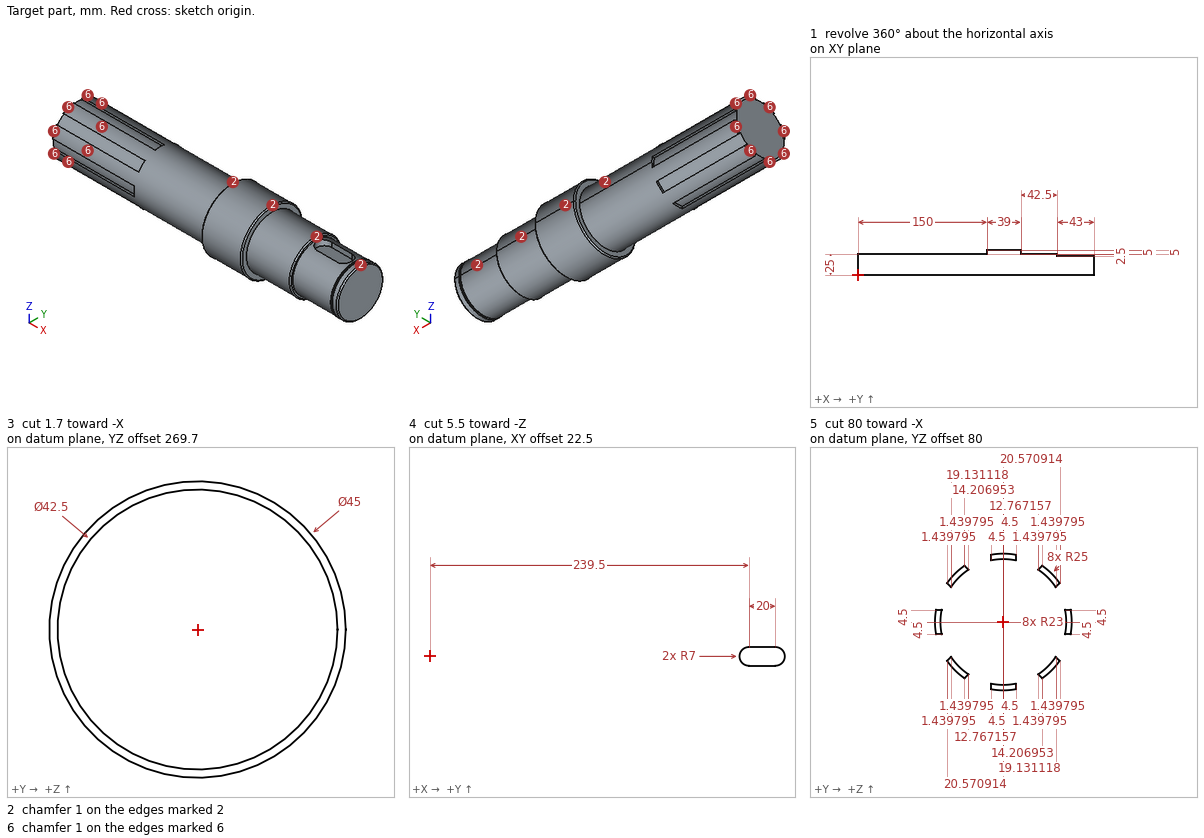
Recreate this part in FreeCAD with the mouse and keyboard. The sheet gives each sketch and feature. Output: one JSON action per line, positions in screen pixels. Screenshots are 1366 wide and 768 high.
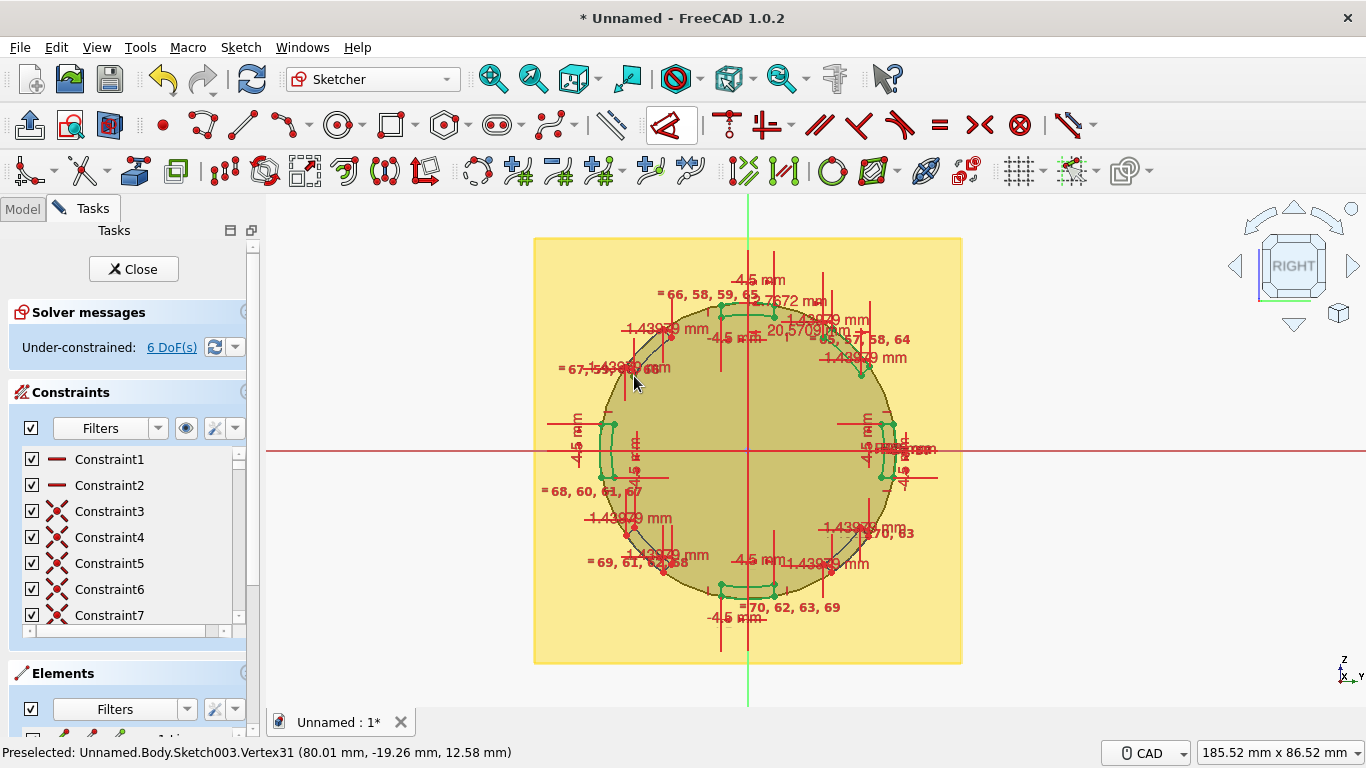
{"action": "left_click", "coordinate": [692, 126]}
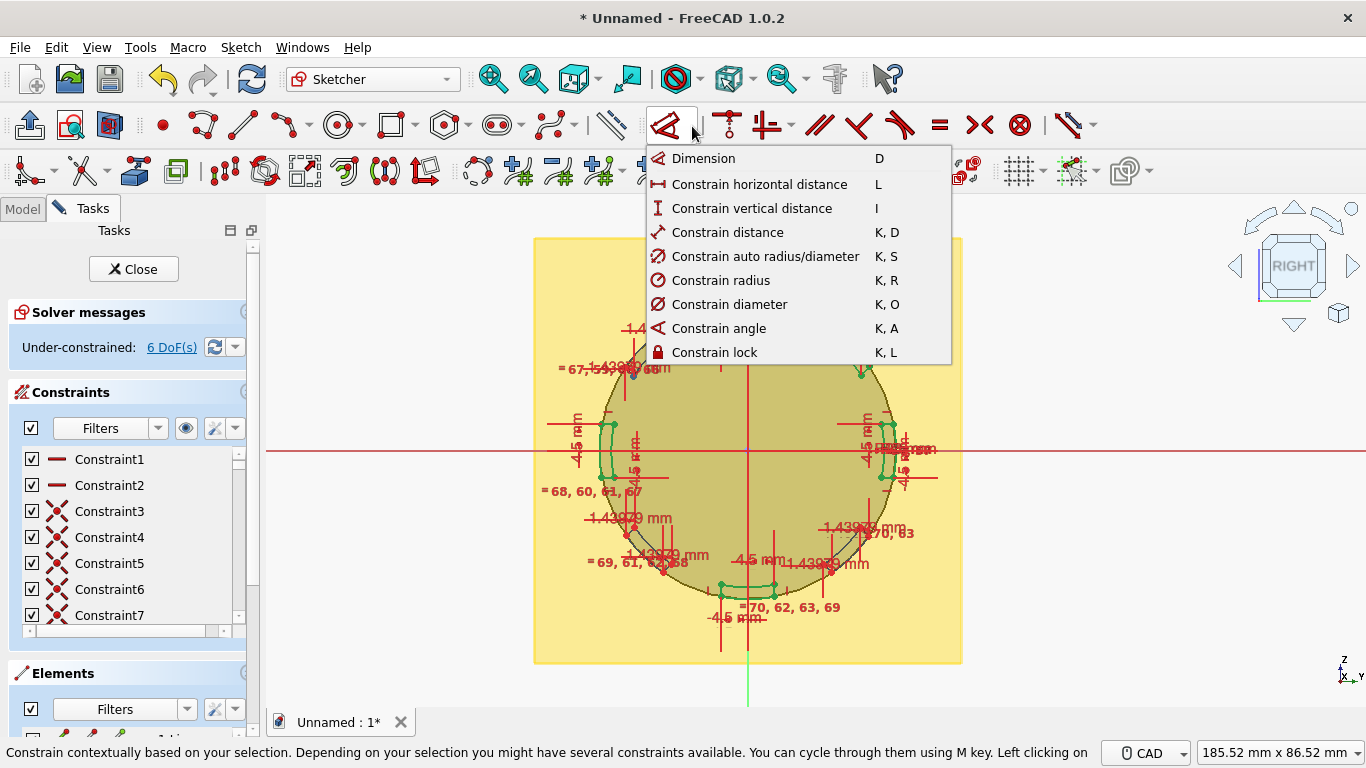
{"action": "left_click", "coordinate": [799, 184]}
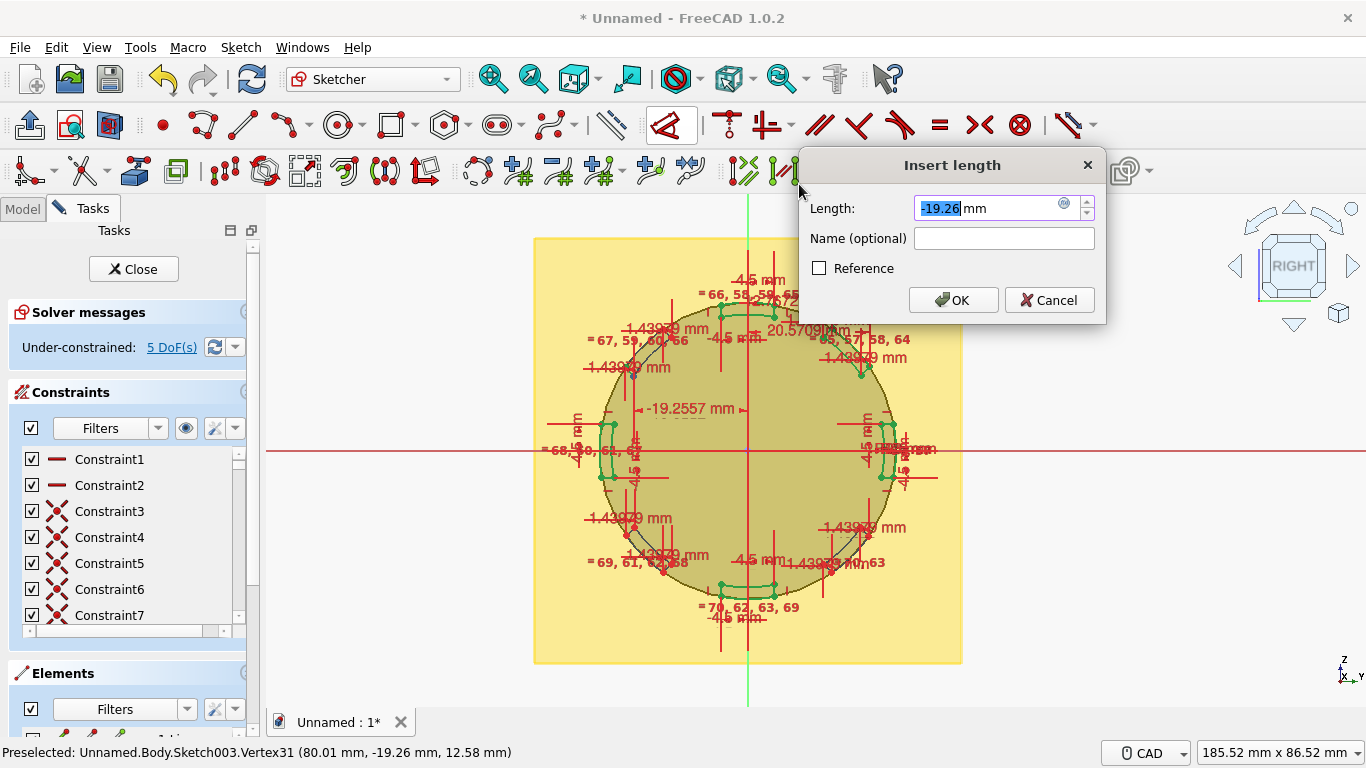
{"action": "type", "text": "-19.131118"}
{"action": "key", "text": "Return"}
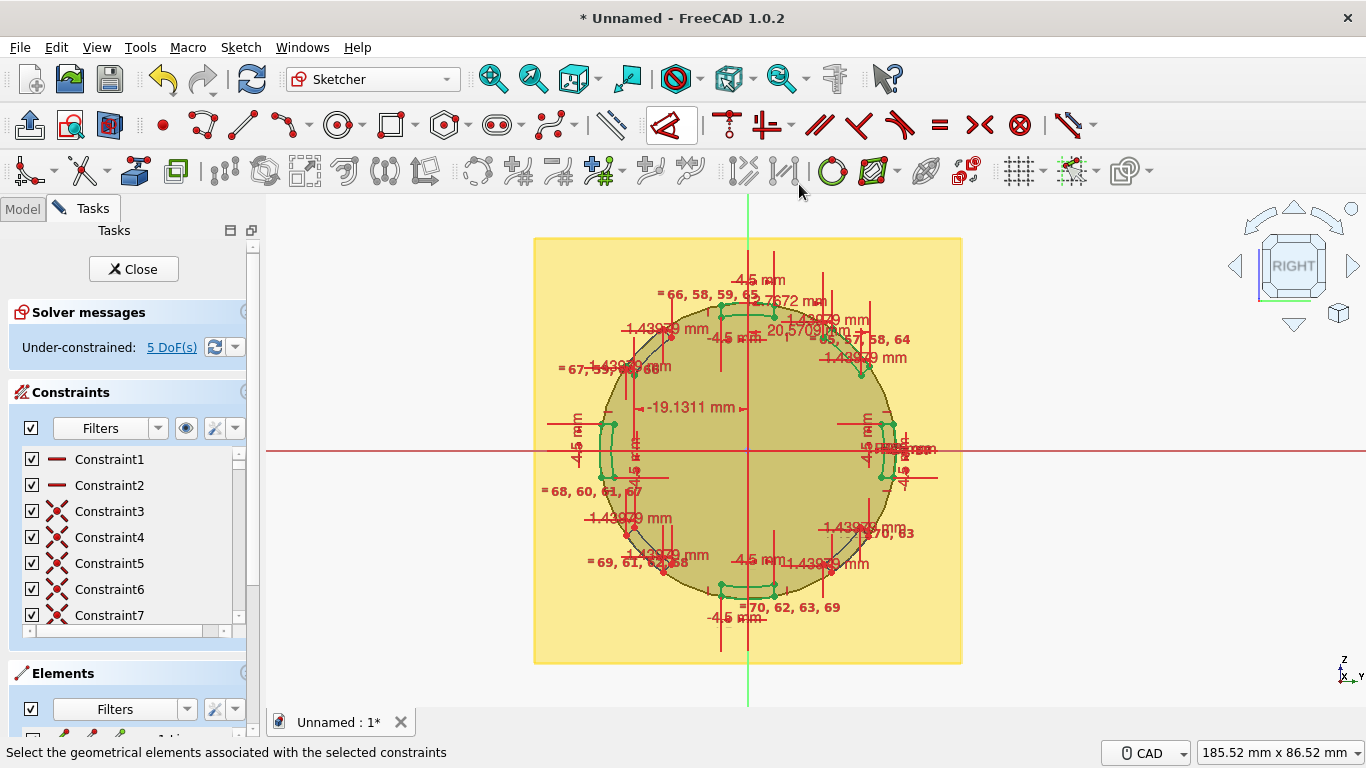
{"action": "left_click", "coordinate": [663, 329]}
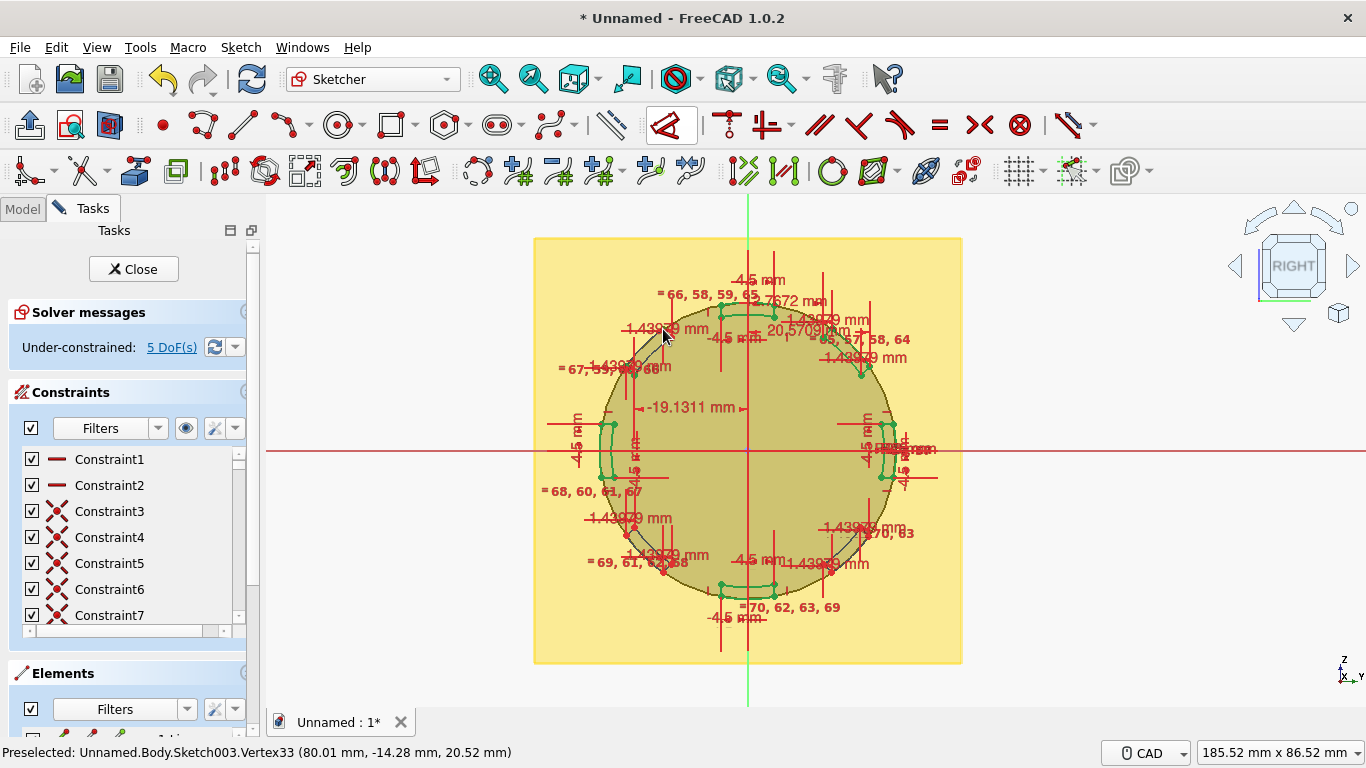
{"action": "key", "text": "l"}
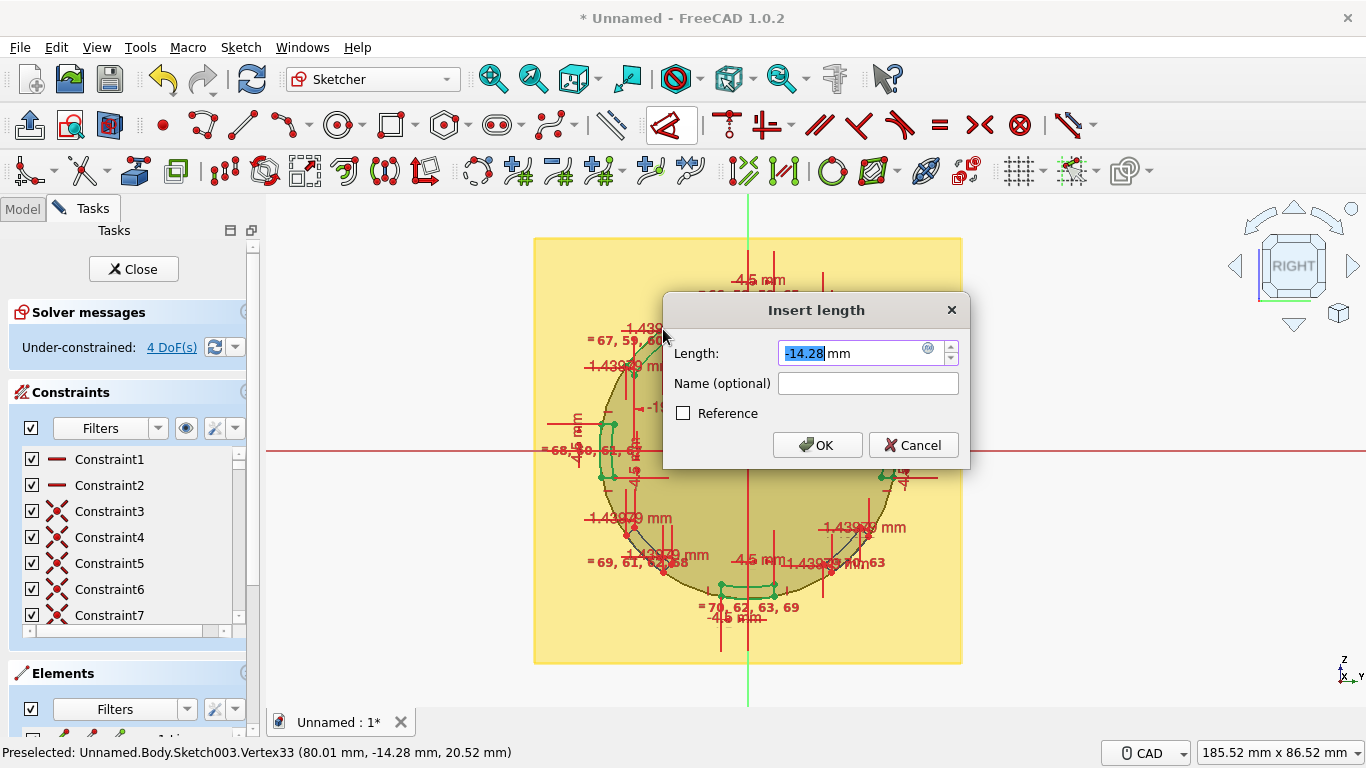
{"action": "type", "text": "-14.206953"}
{"action": "key", "text": "Return"}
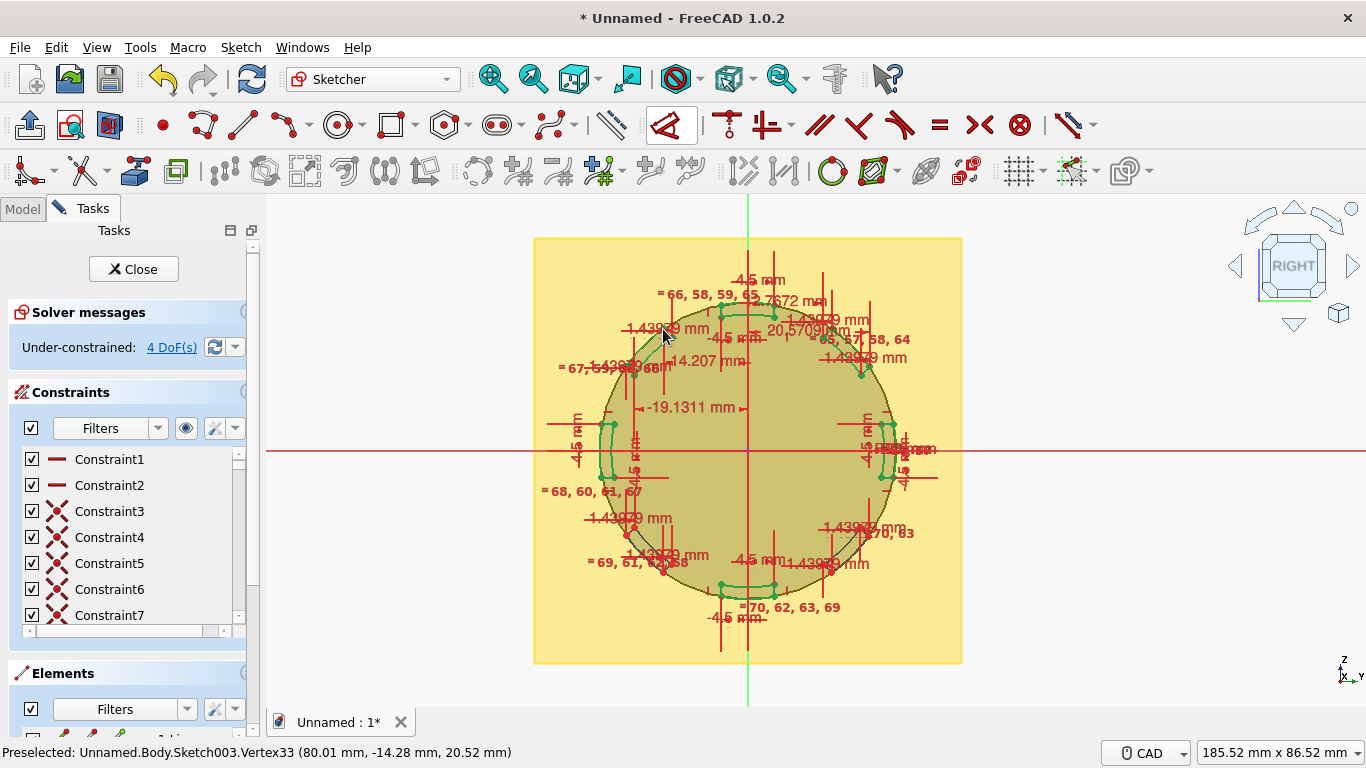
{"action": "left_click", "coordinate": [672, 564]}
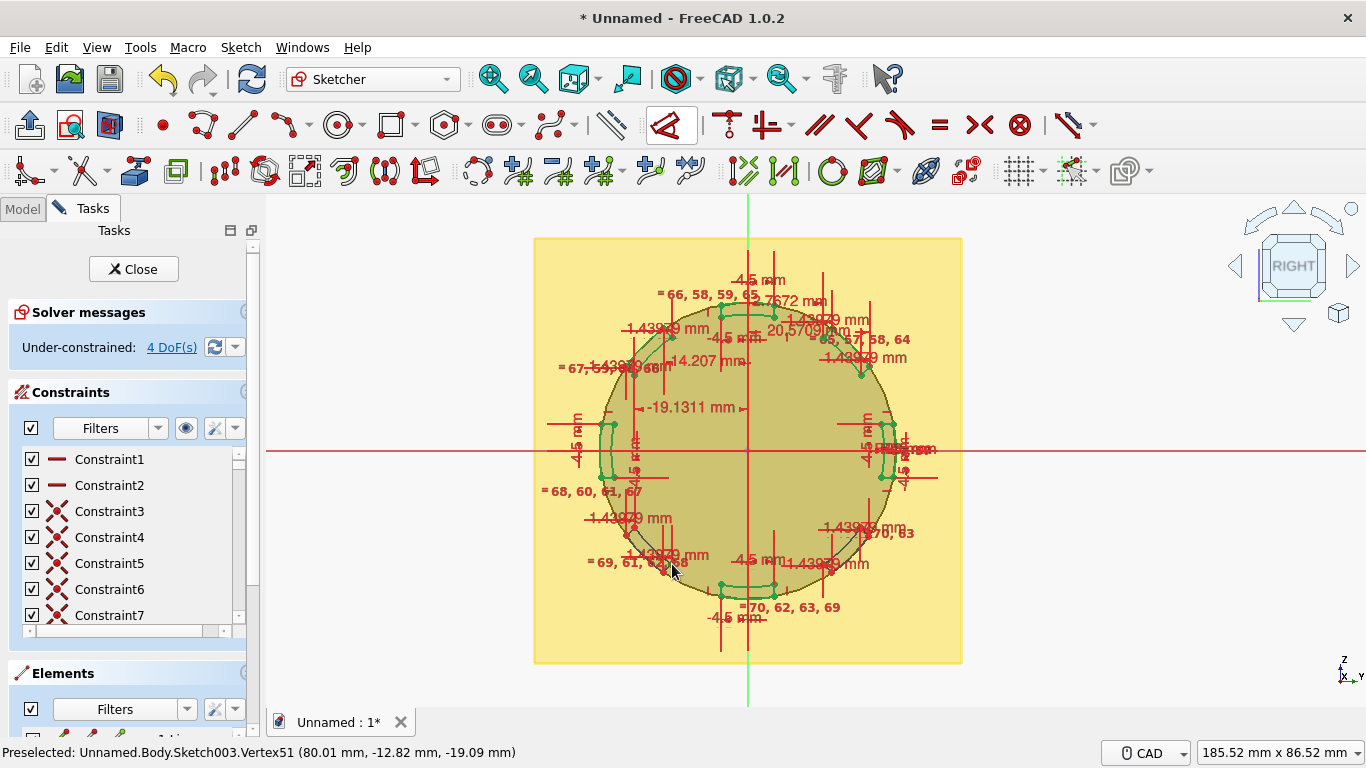
{"action": "key", "text": "l"}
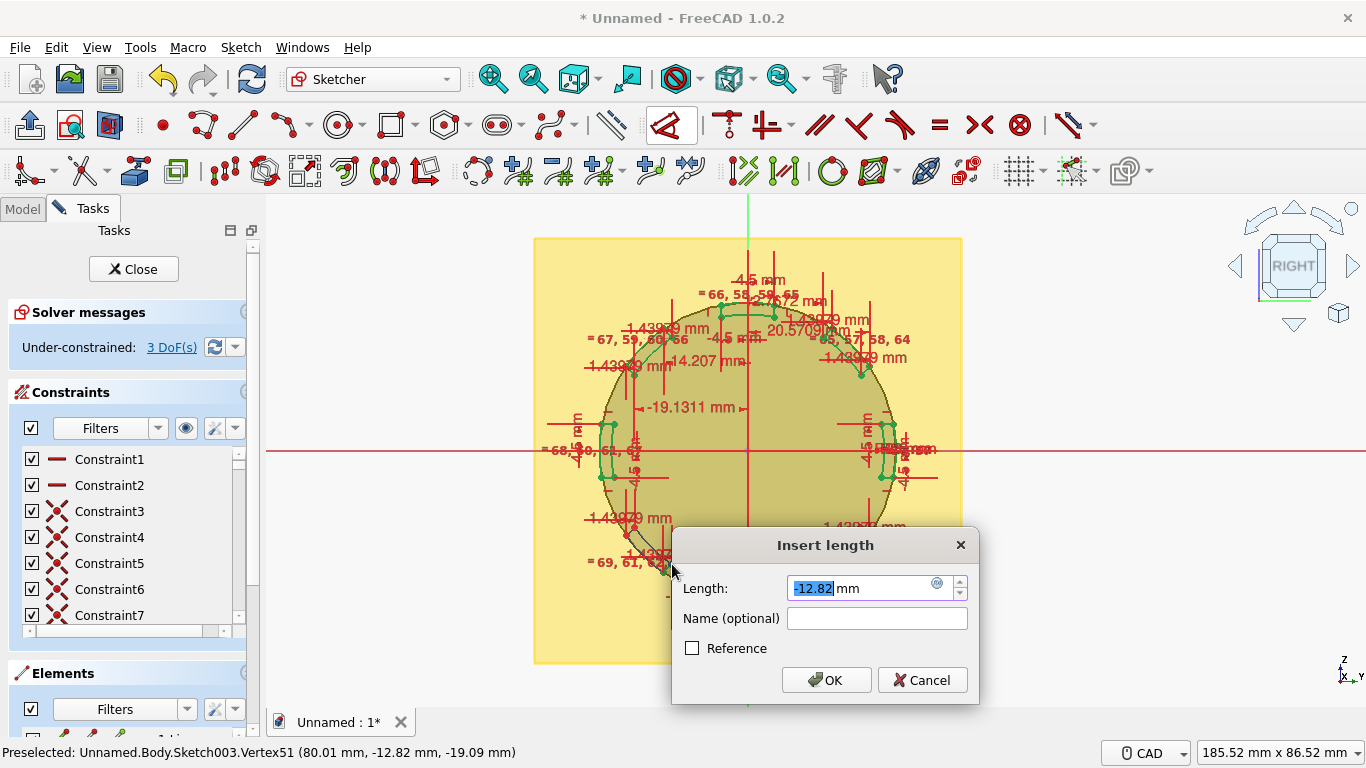
{"action": "type", "text": "-12.767157"}
{"action": "key", "text": "Return"}